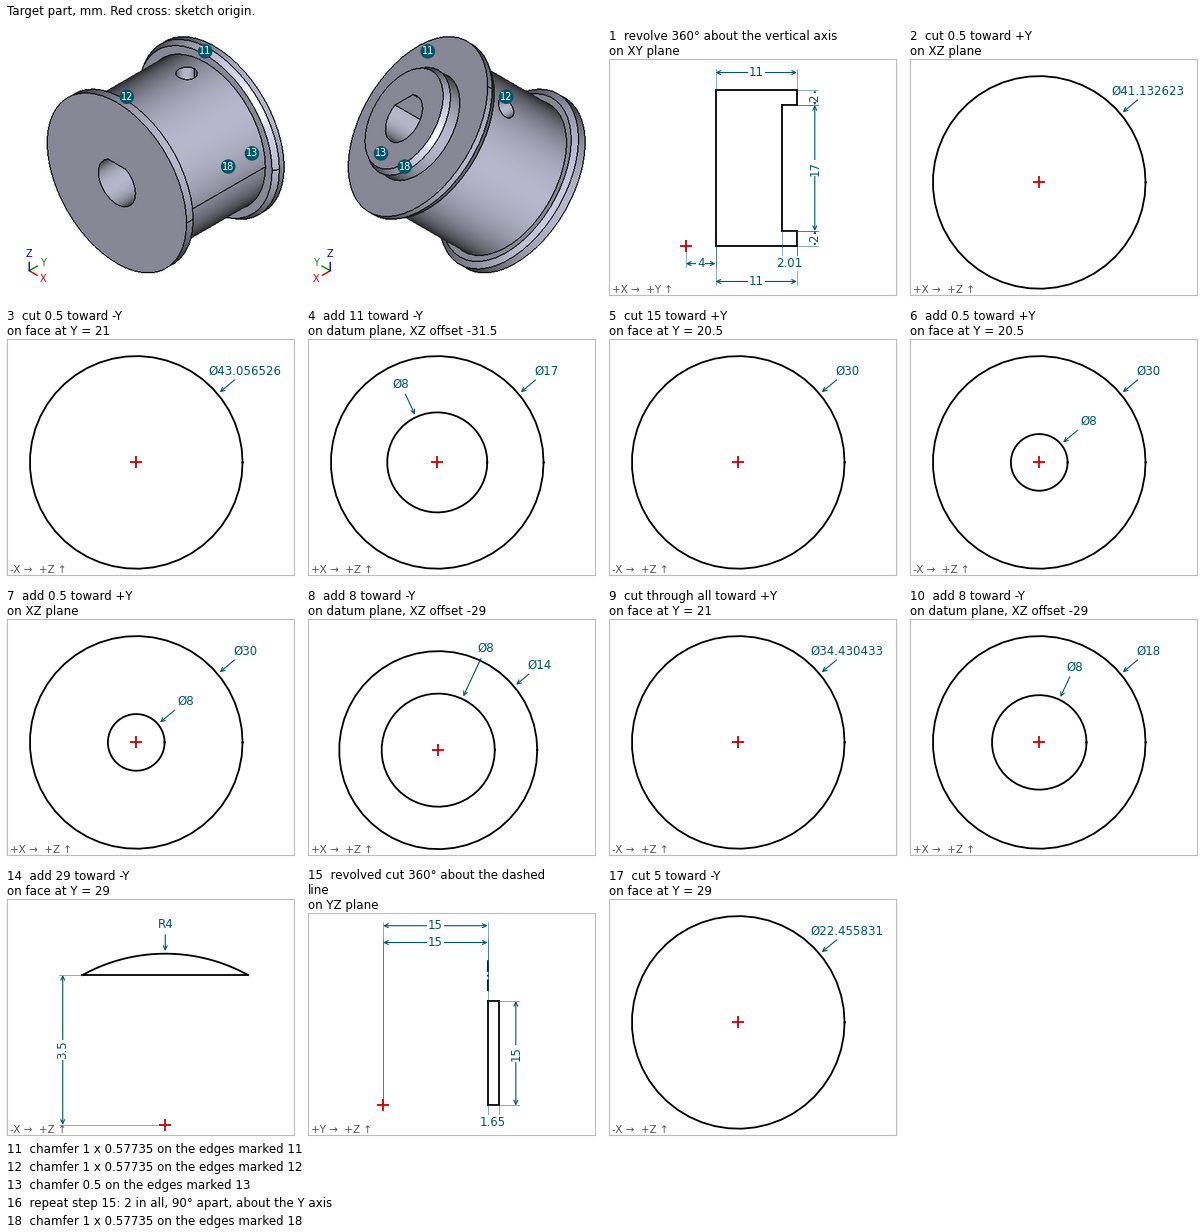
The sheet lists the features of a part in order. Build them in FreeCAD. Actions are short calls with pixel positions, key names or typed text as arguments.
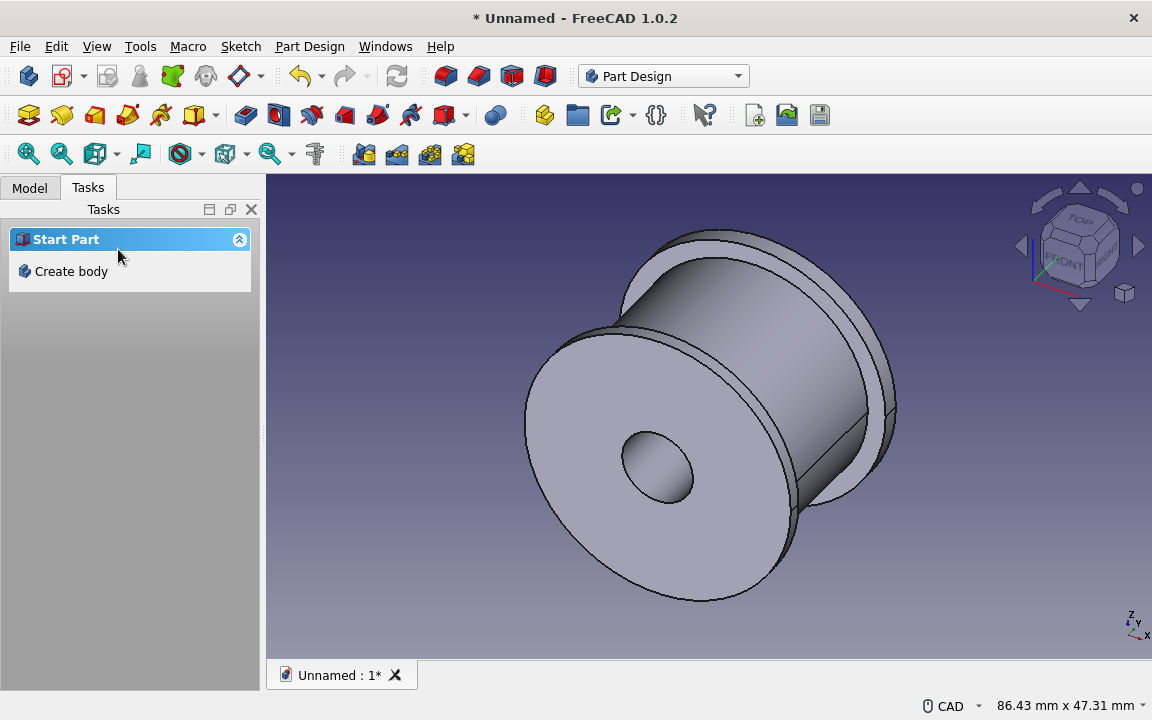
key(4)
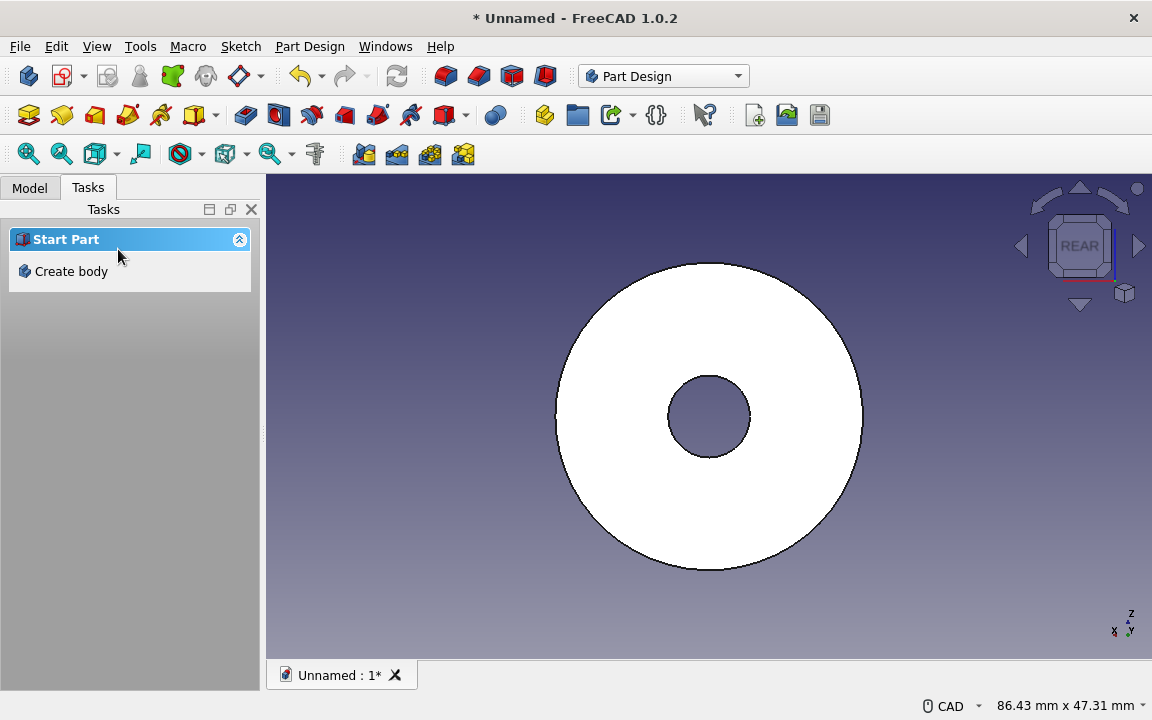
click(665, 503)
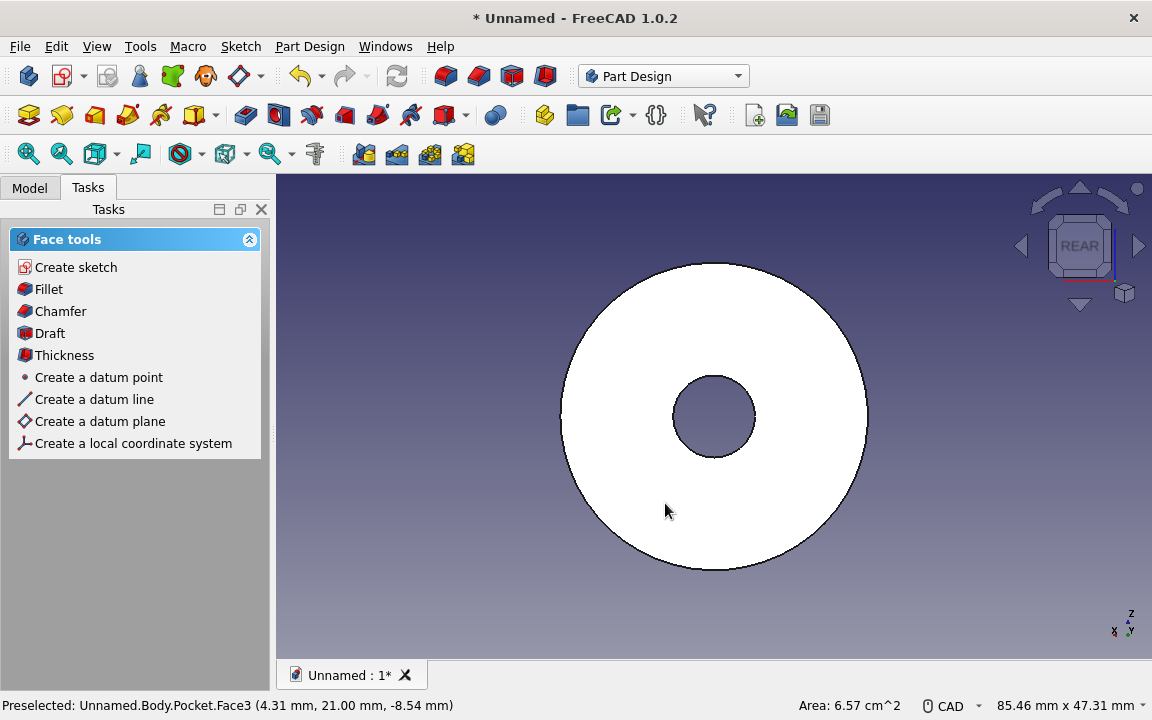
click(62, 76)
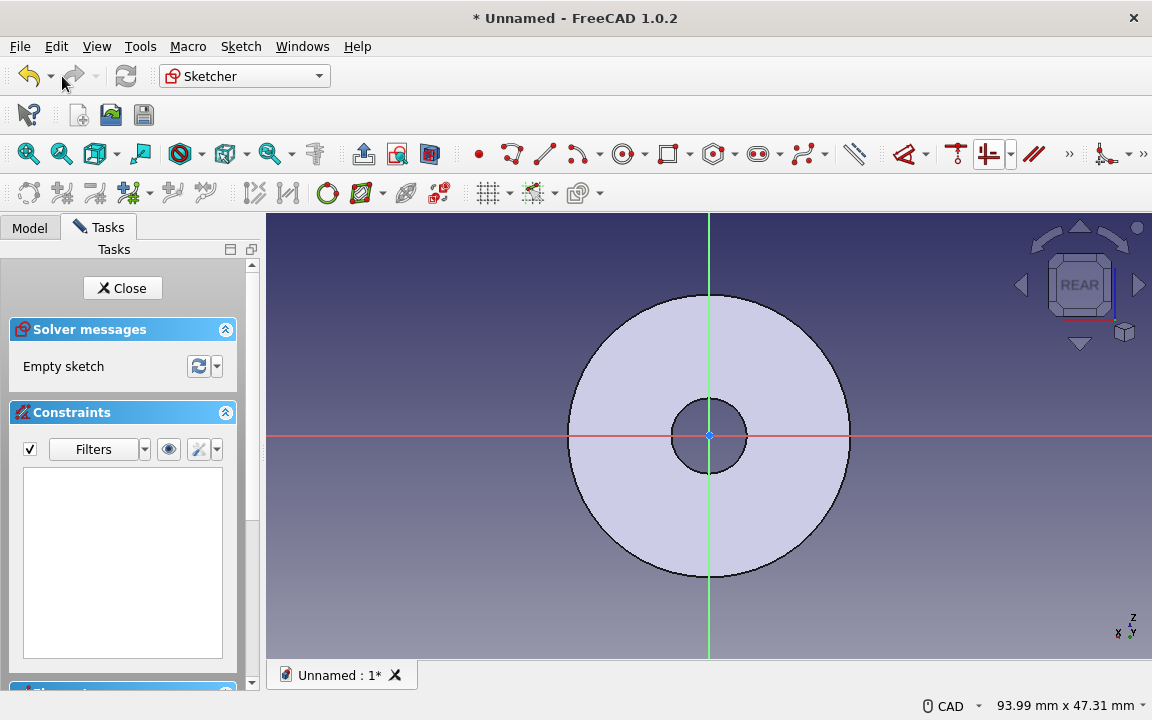
scroll(501, 436, down, 2)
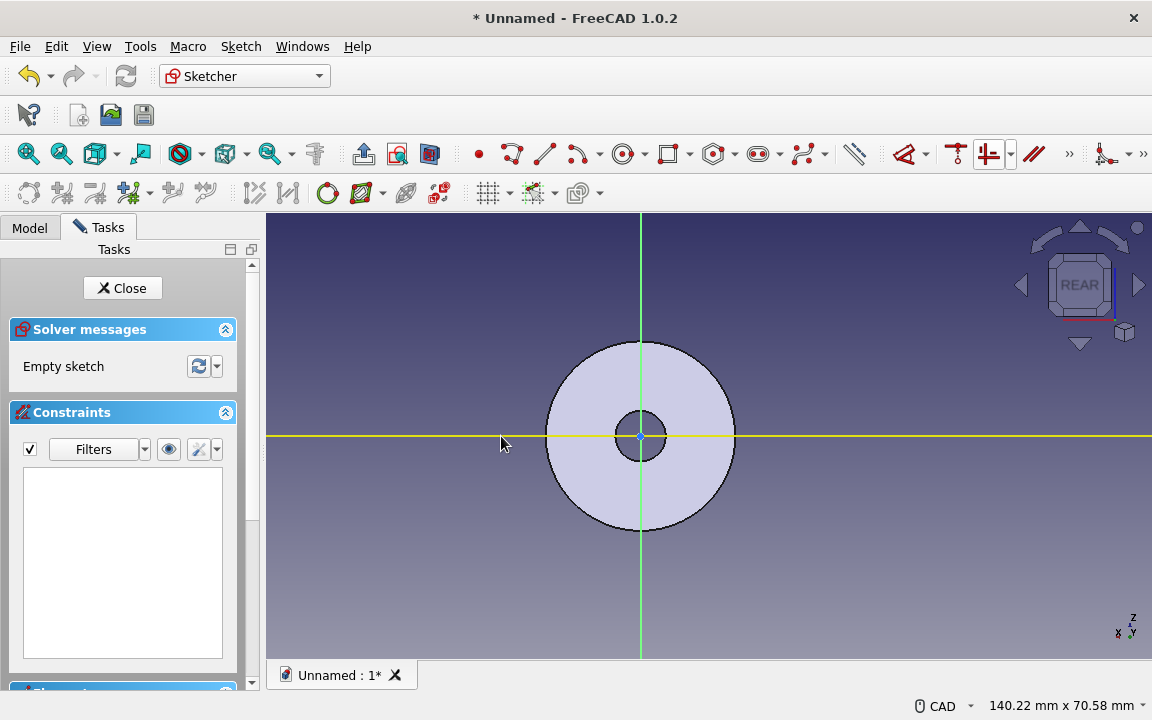
click(622, 154)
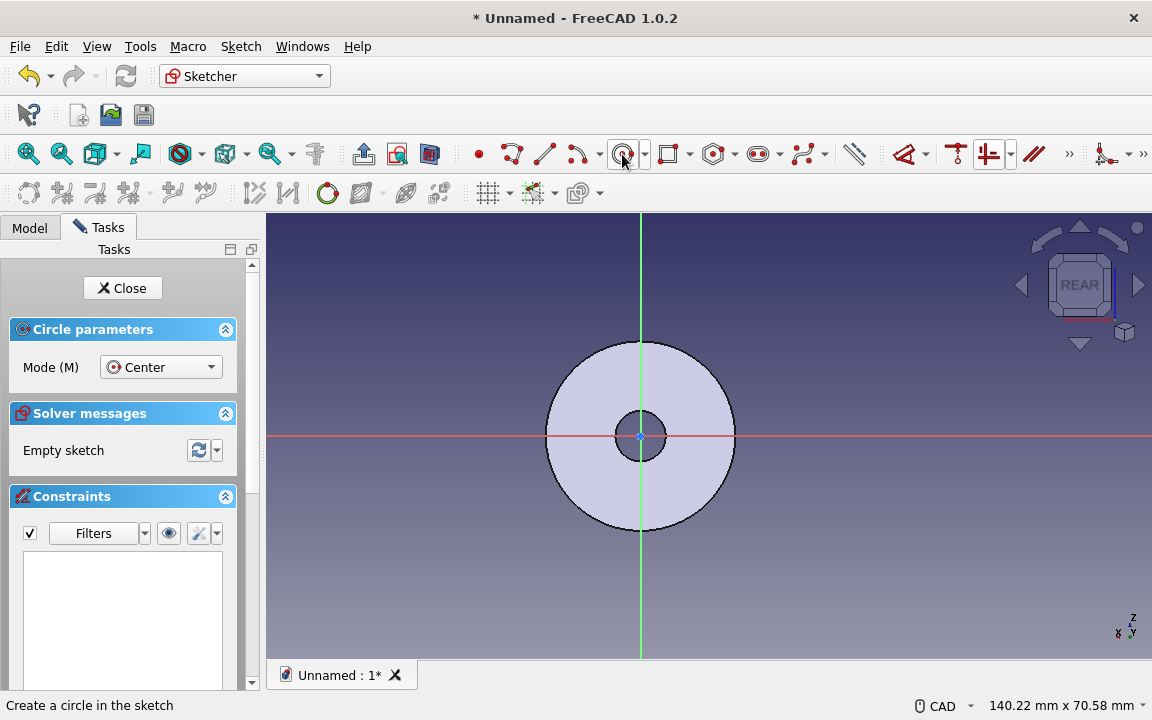
click(641, 436)
move(737, 340)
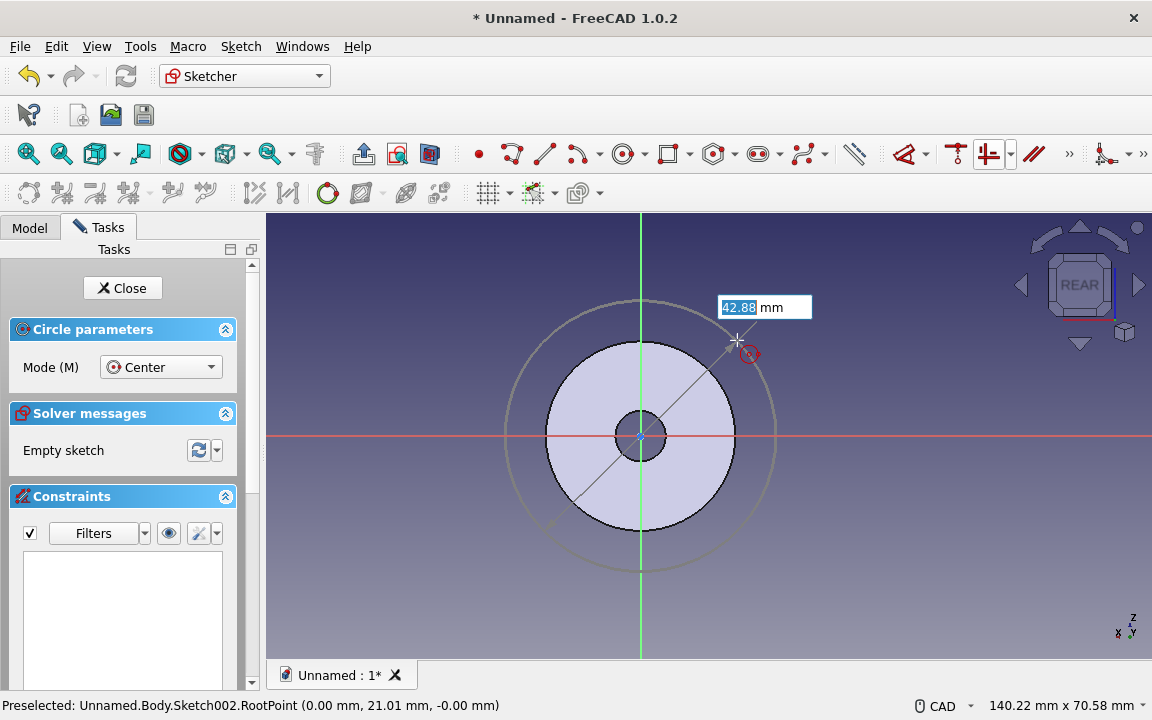
text(43.056526)
key(Return)
key(Escape)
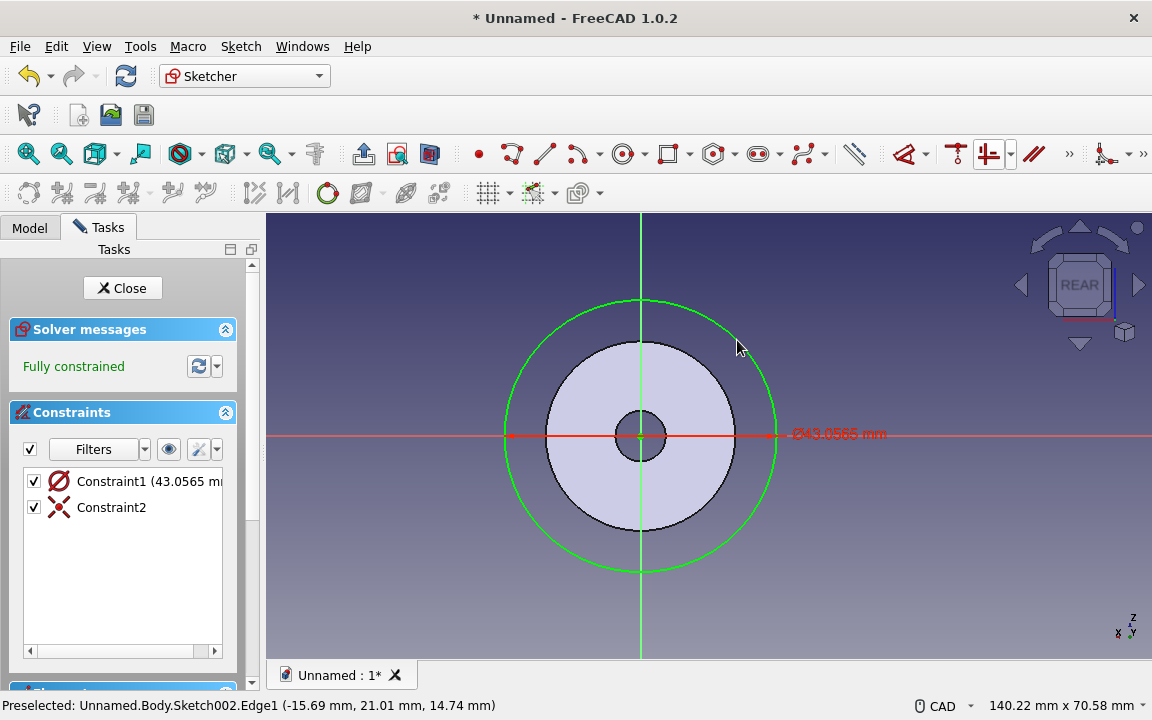
click(123, 288)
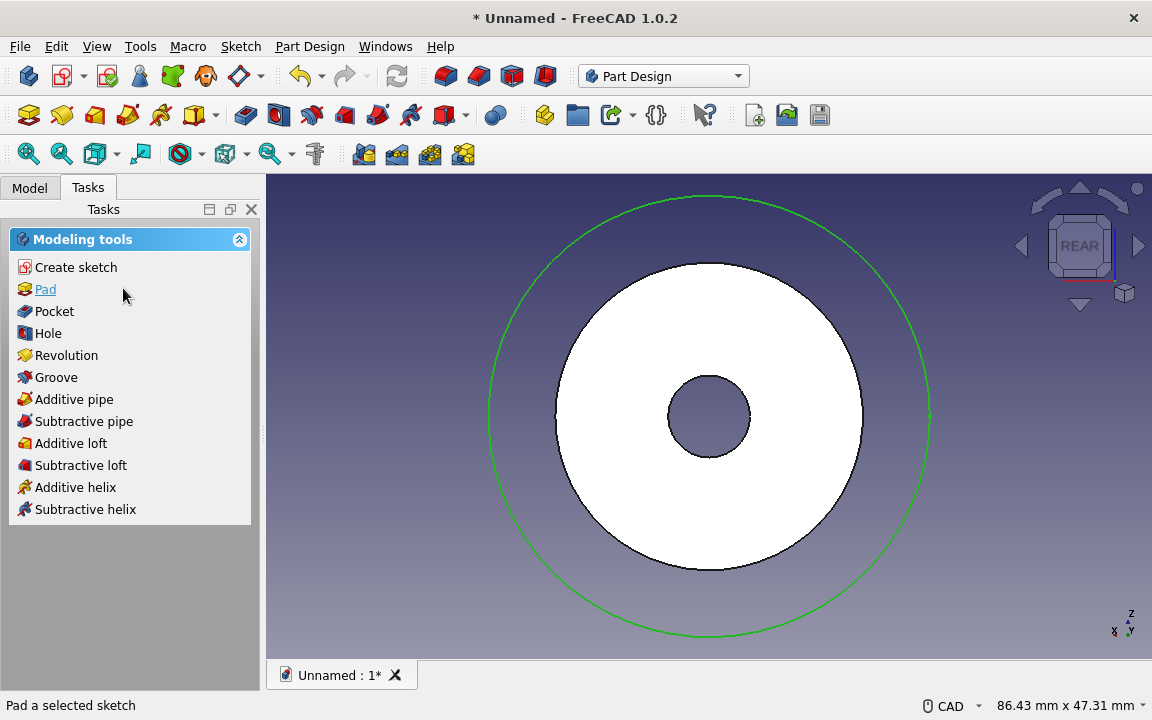
click(246, 116)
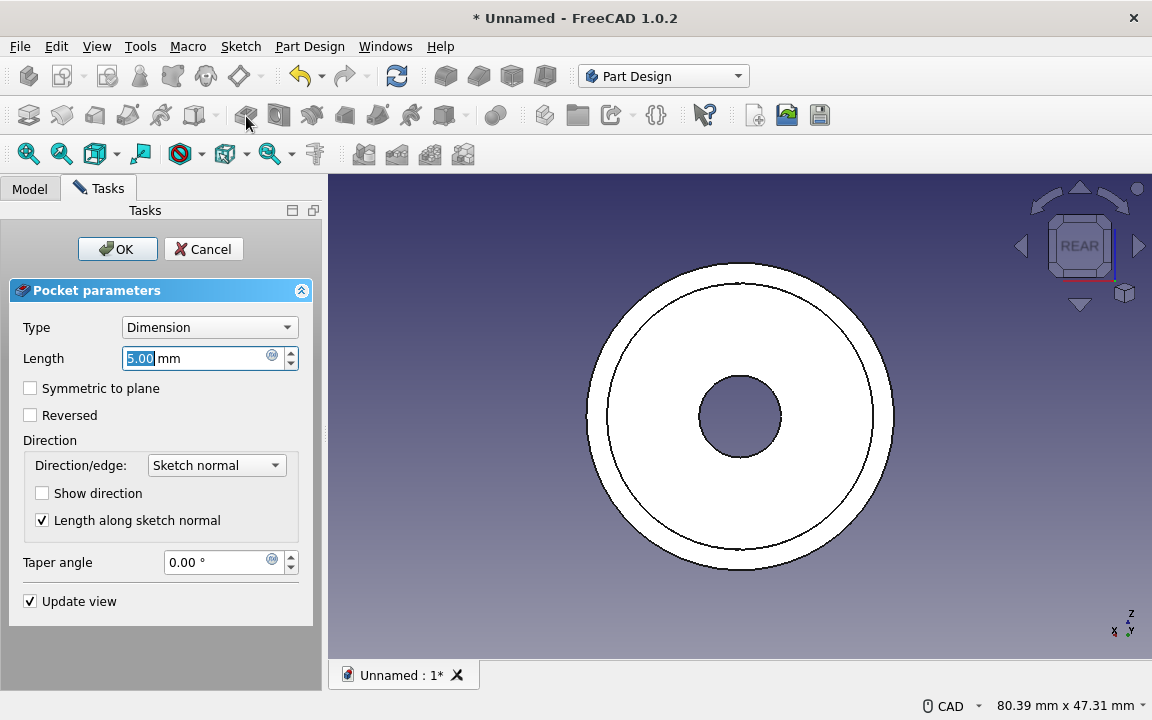
text(0.5)
key(Tab)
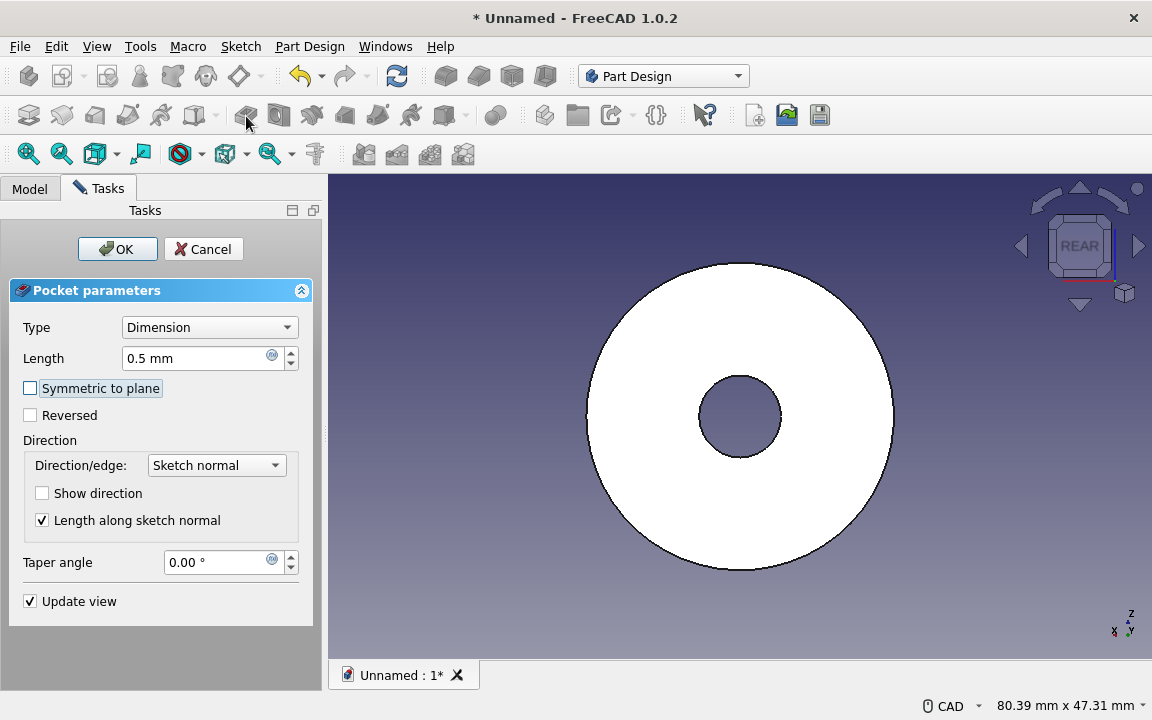
click(118, 249)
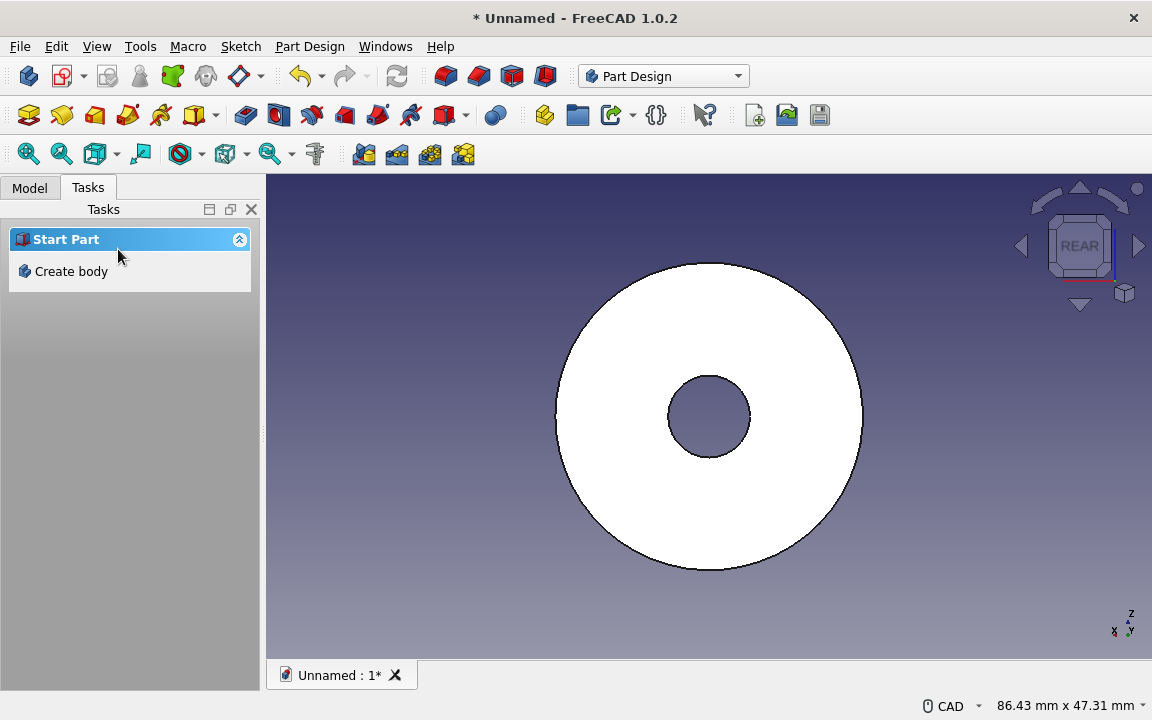
click(30, 188)